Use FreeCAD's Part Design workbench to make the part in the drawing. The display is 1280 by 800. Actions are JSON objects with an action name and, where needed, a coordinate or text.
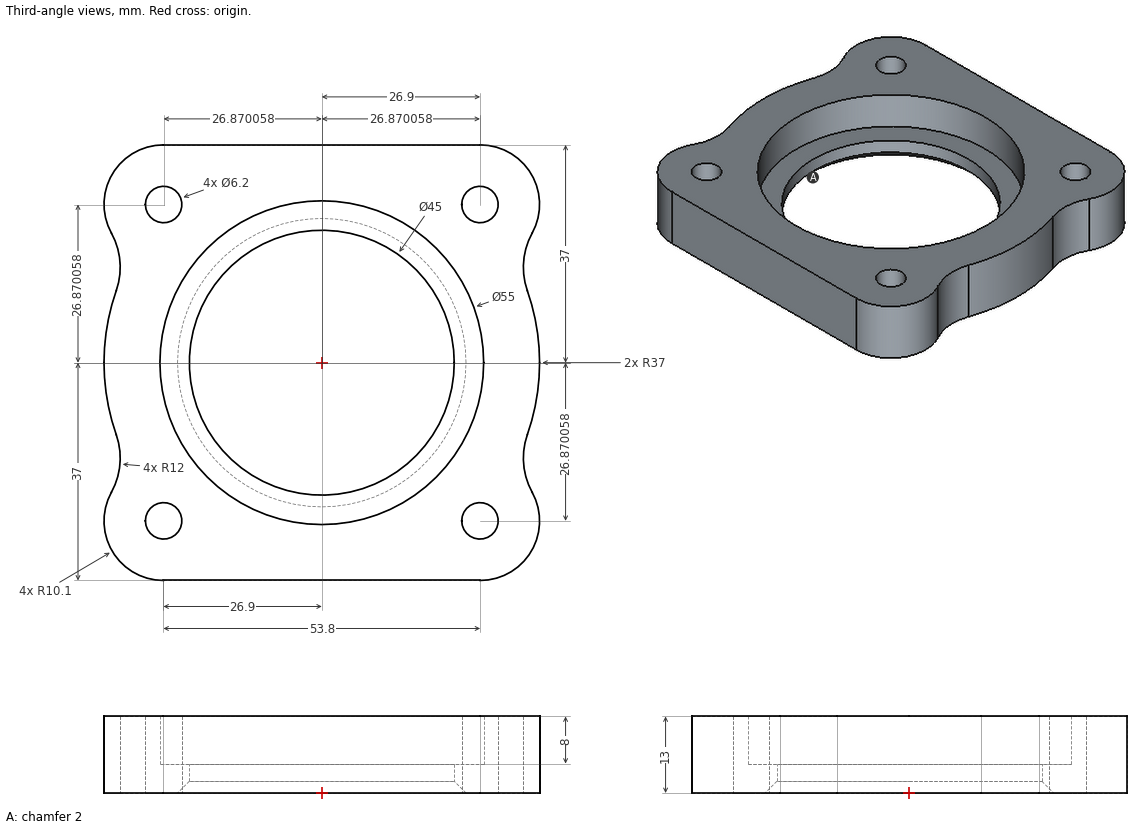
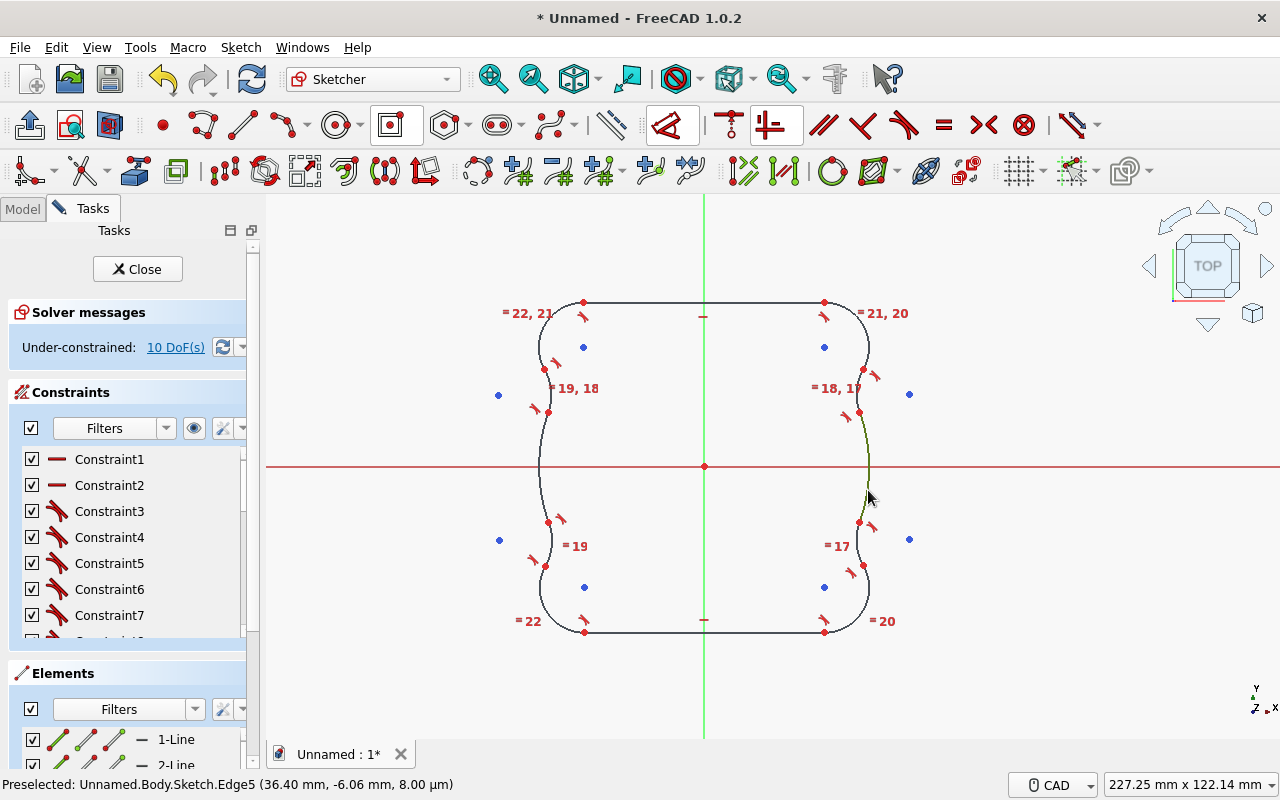
{"action": "left_click", "coordinate": [541, 445]}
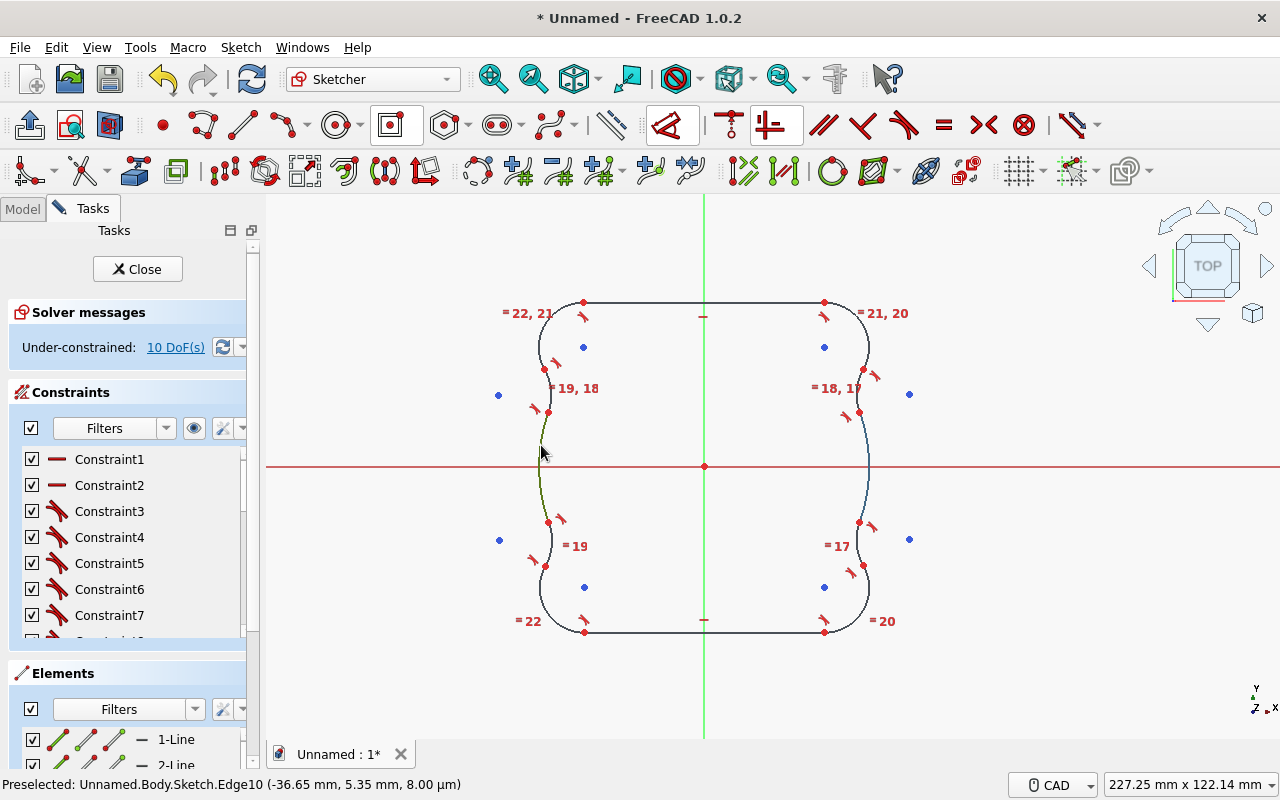
{"action": "key", "text": "e"}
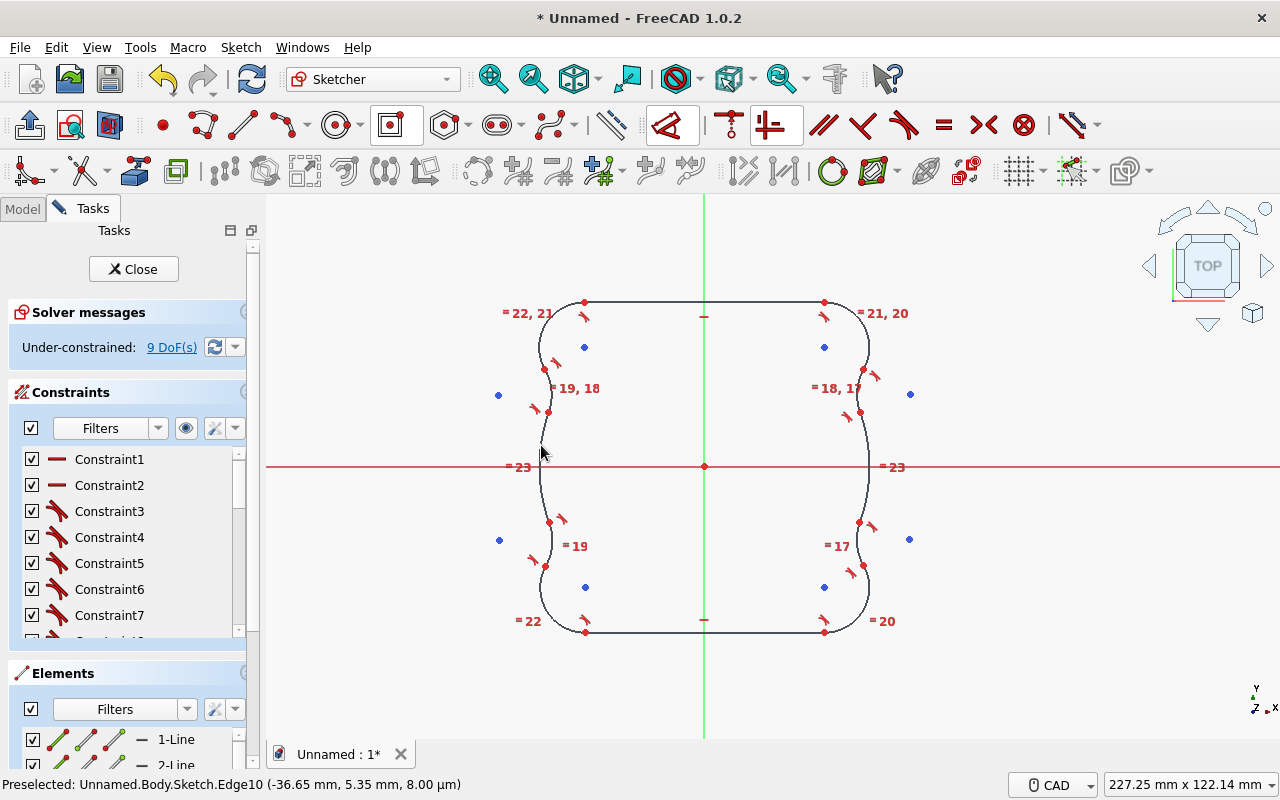
{"action": "left_click", "coordinate": [666, 126]}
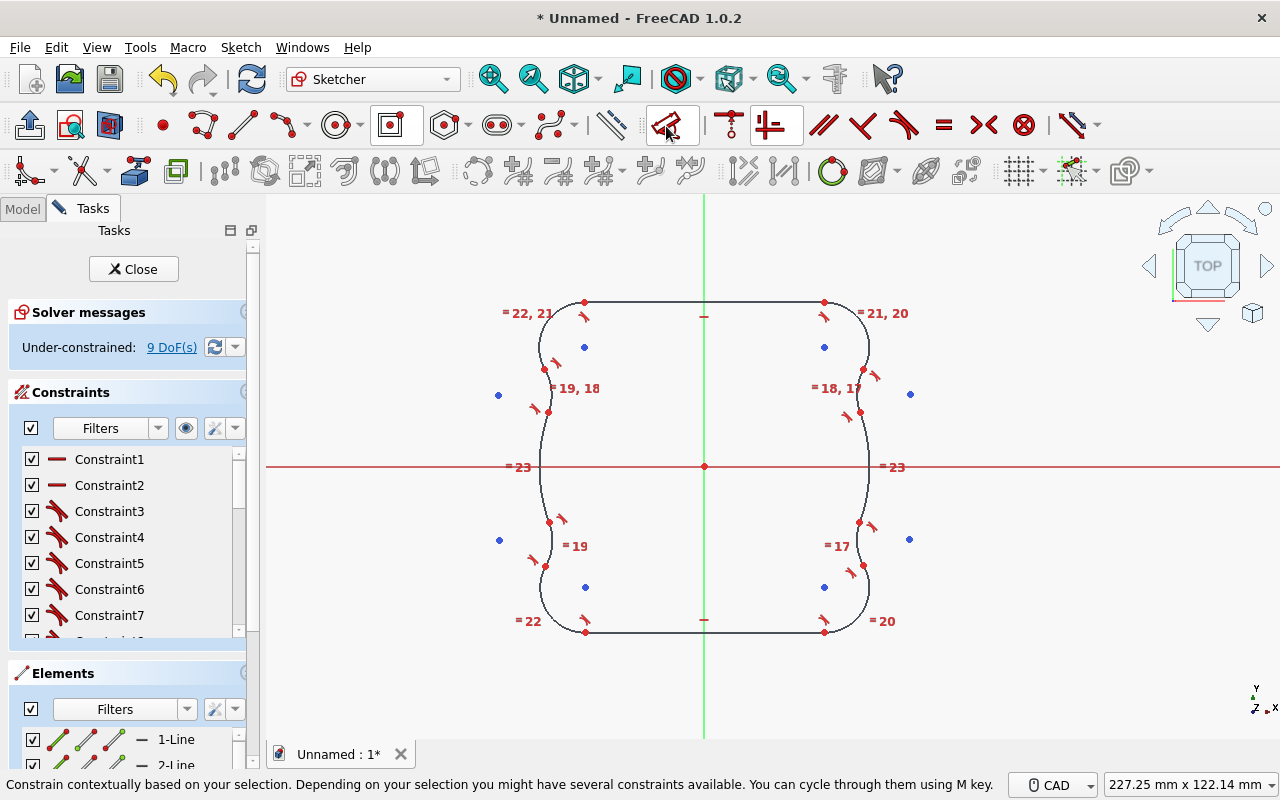
{"action": "left_click", "coordinate": [851, 624]}
{"action": "left_click", "coordinate": [870, 650]}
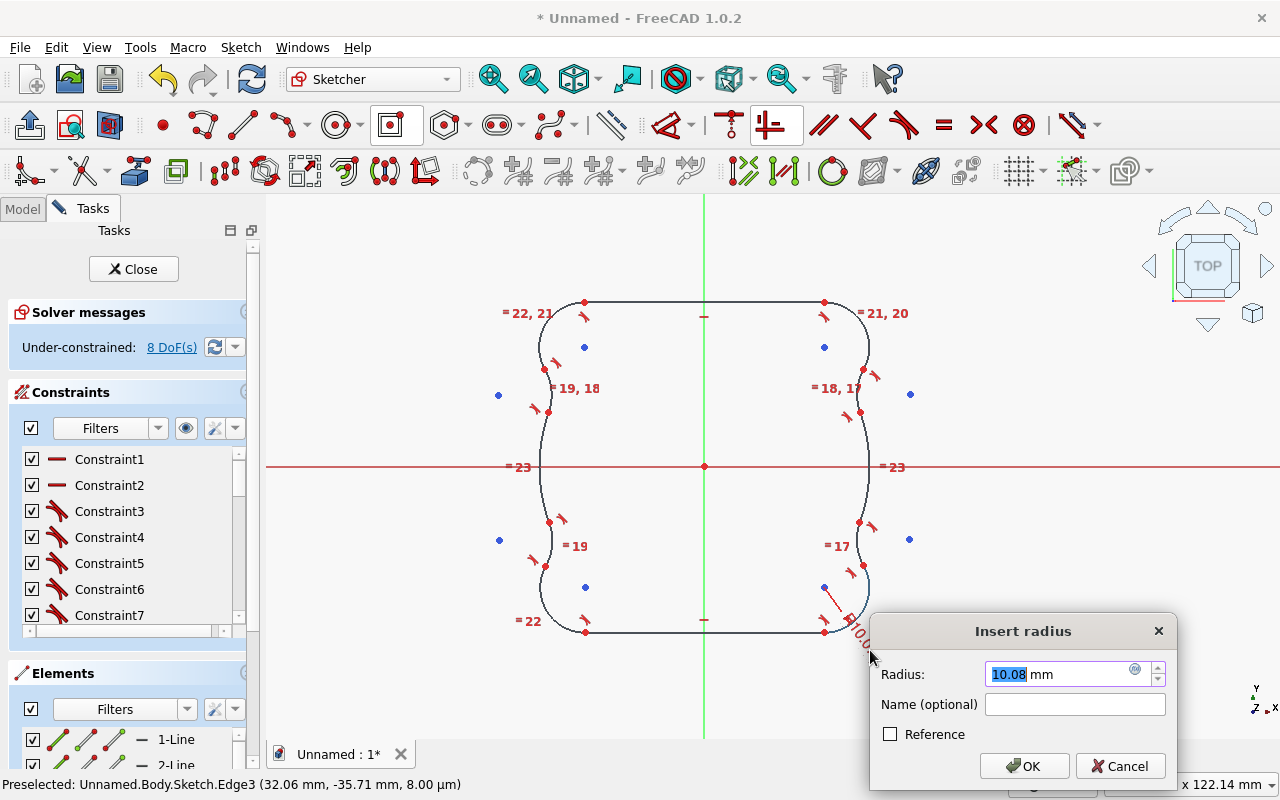
{"action": "type", "text": "10.1"}
{"action": "key", "text": "Return"}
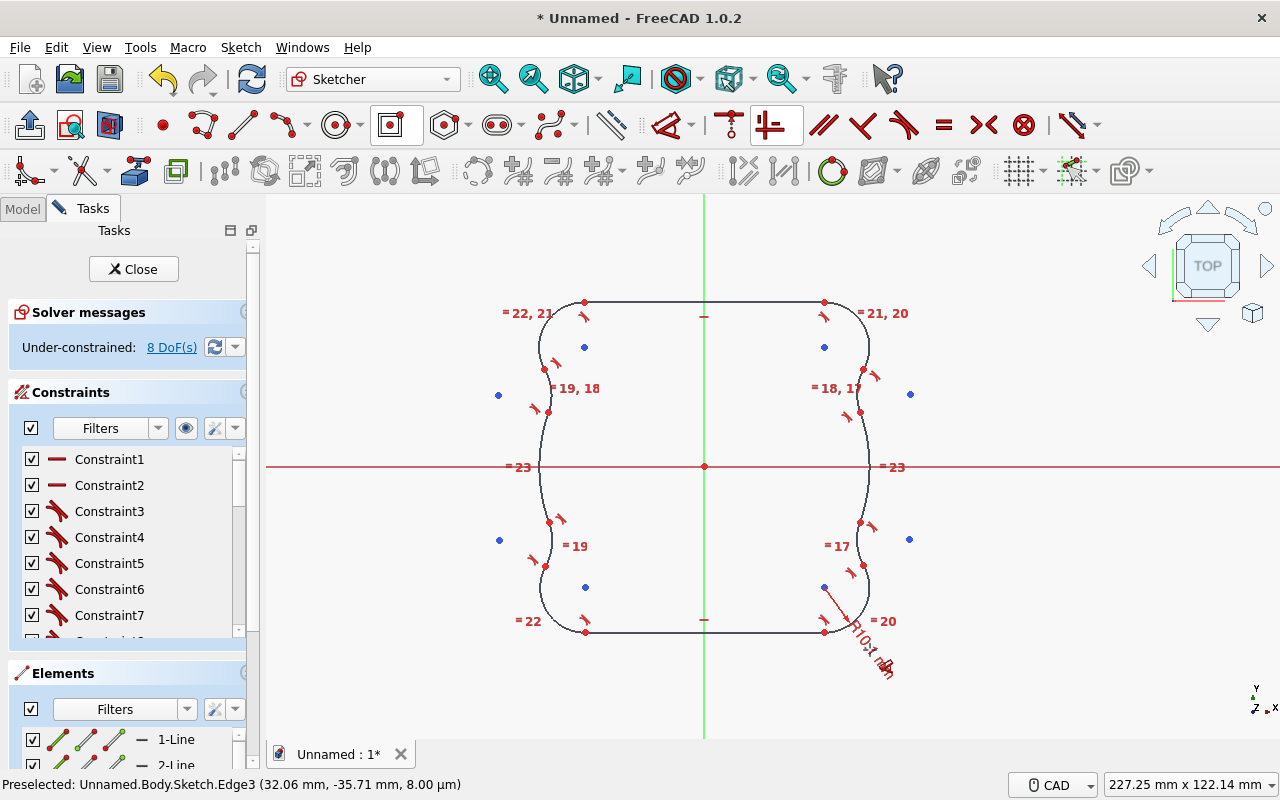
{"action": "left_click", "coordinate": [857, 535]}
{"action": "left_click", "coordinate": [825, 532]}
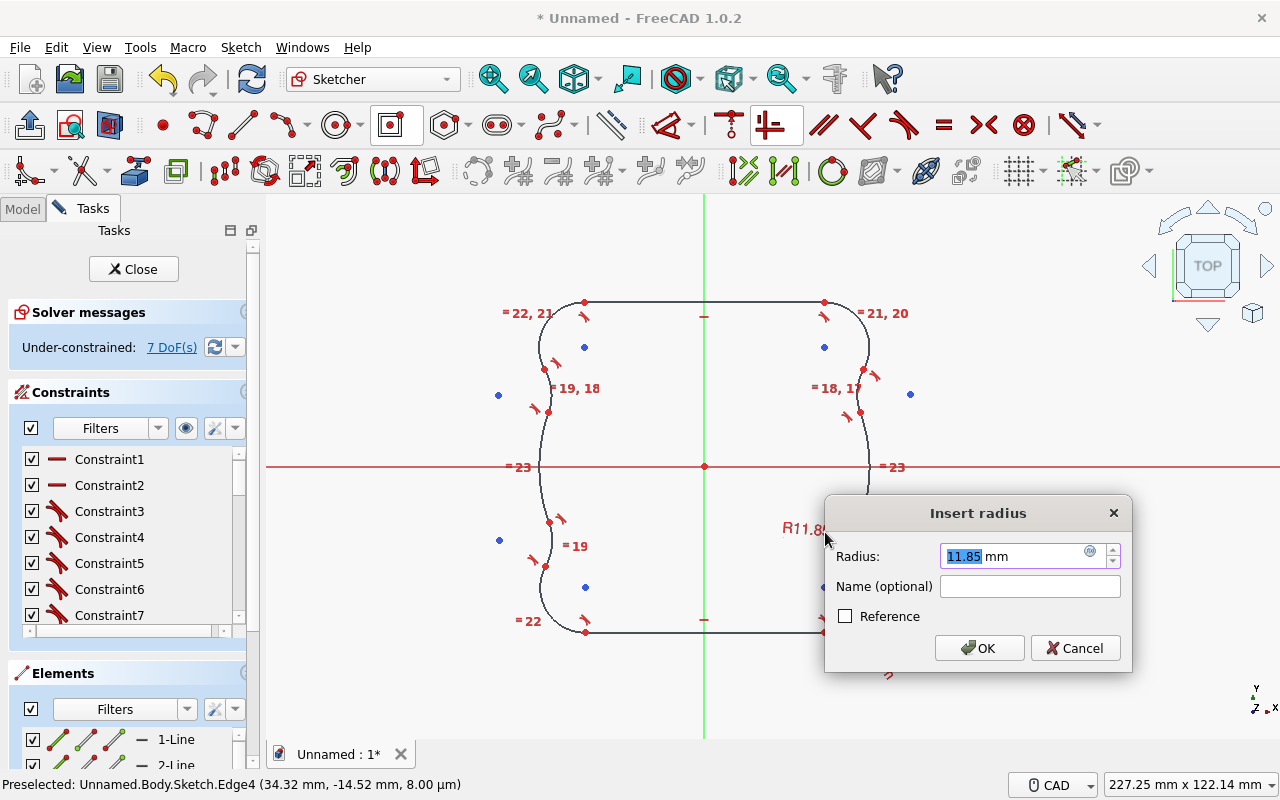
{"action": "type", "text": "12"}
{"action": "key", "text": "Return"}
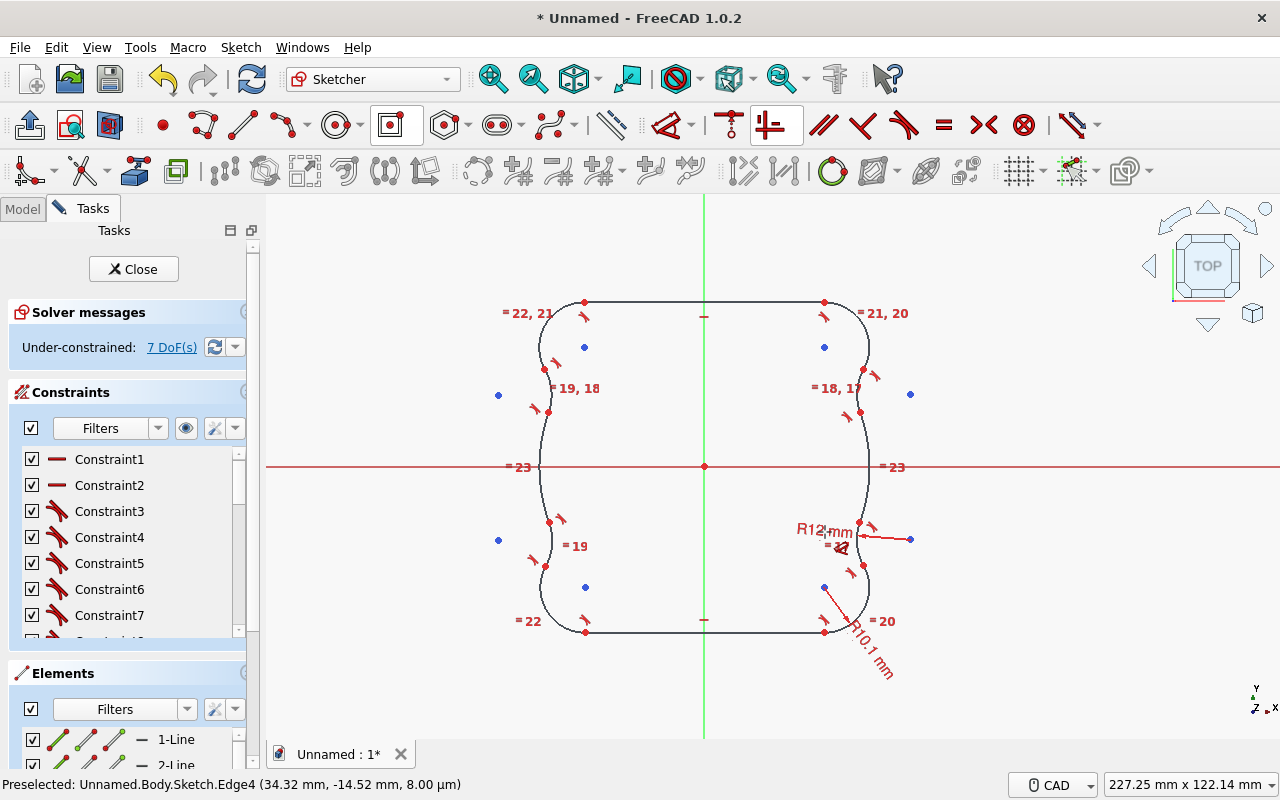
{"action": "left_click", "coordinate": [868, 490]}
{"action": "left_click", "coordinate": [900, 494]}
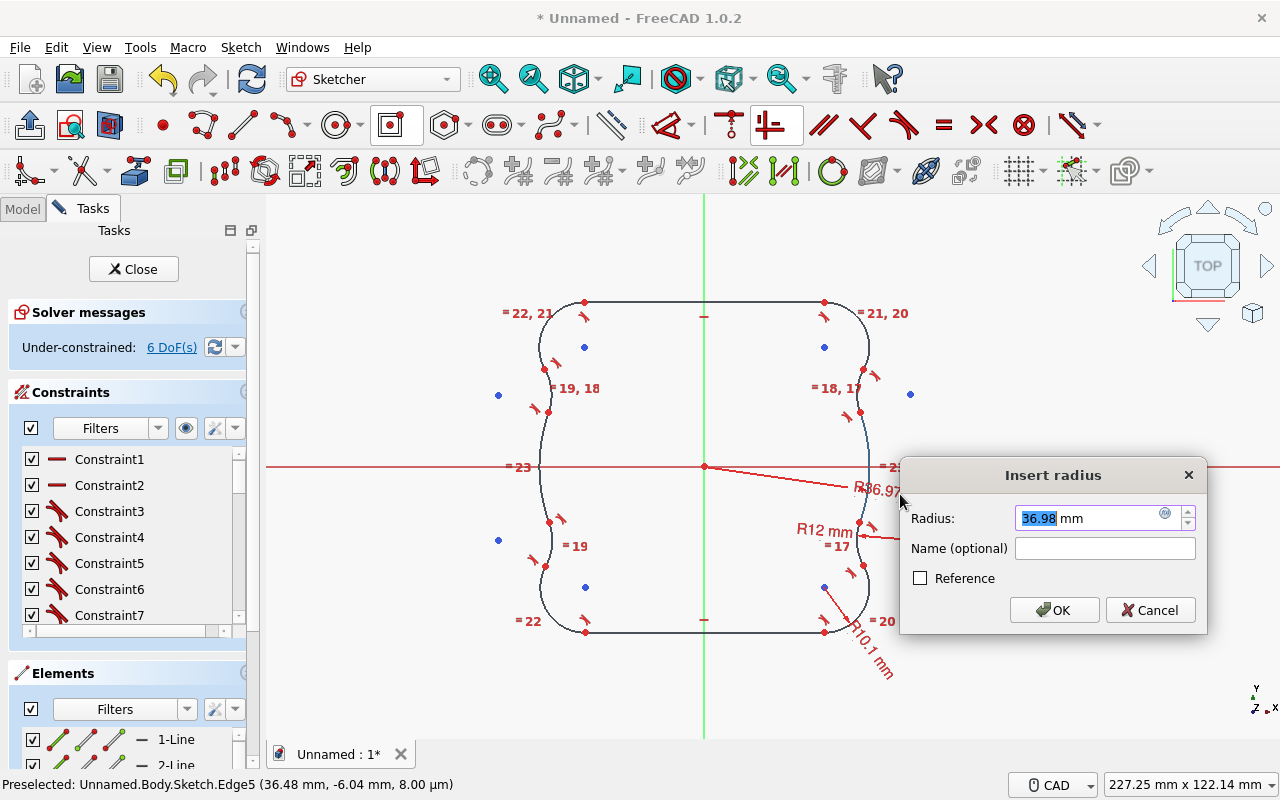
{"action": "type", "text": "37"}
{"action": "key", "text": "Return"}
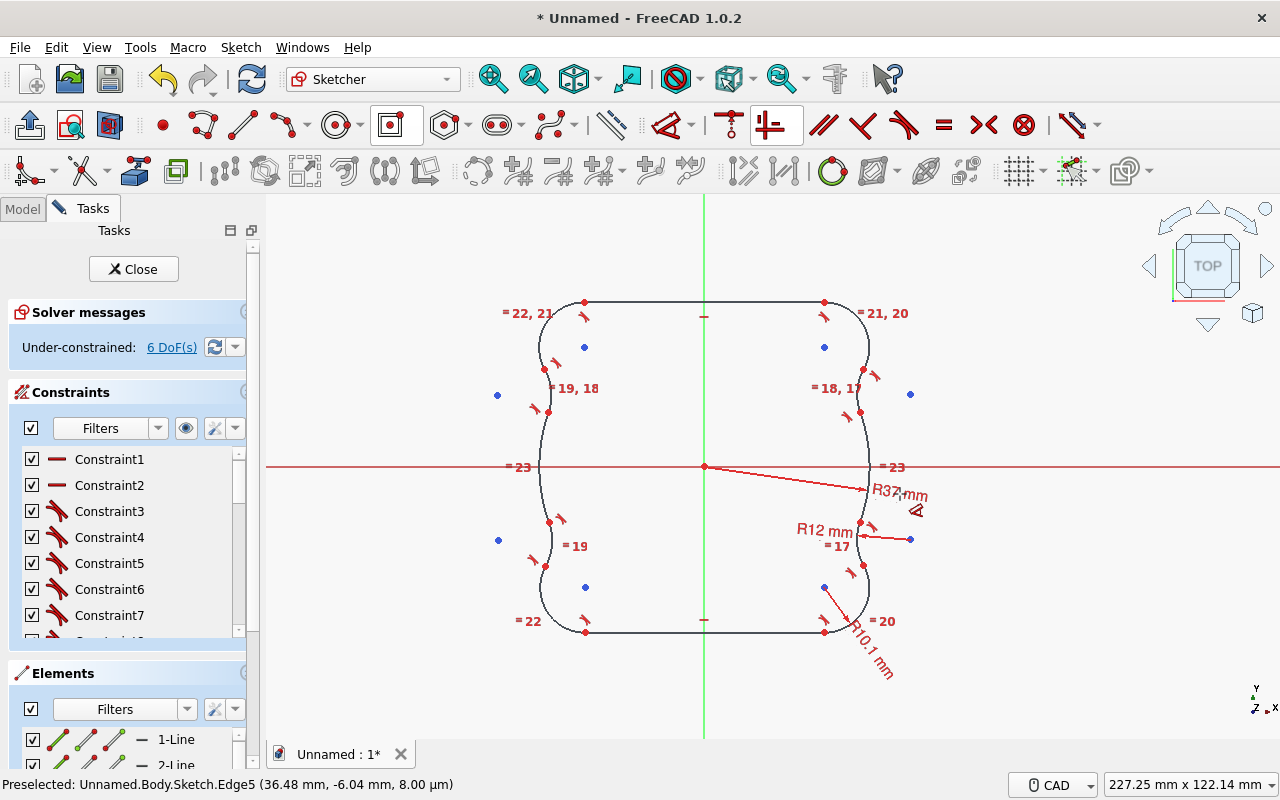
{"action": "left_click", "coordinate": [585, 633]}
{"action": "left_click", "coordinate": [738, 550]}